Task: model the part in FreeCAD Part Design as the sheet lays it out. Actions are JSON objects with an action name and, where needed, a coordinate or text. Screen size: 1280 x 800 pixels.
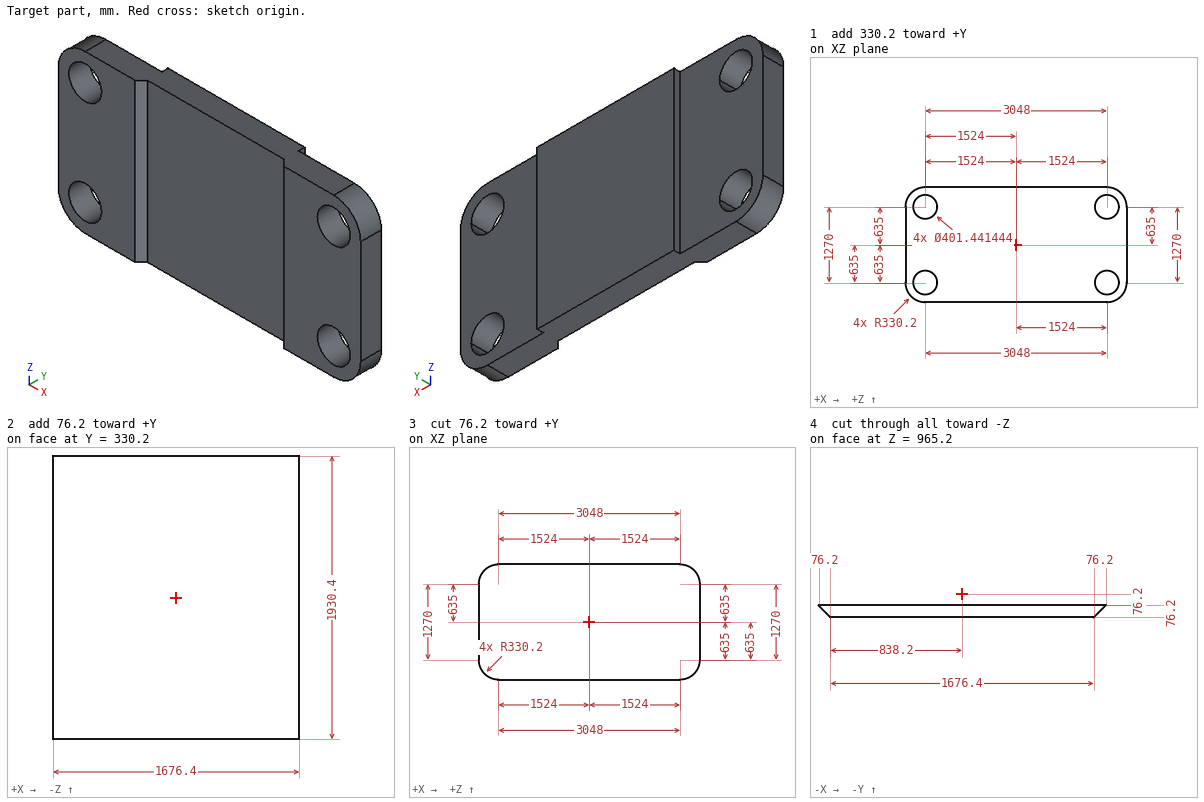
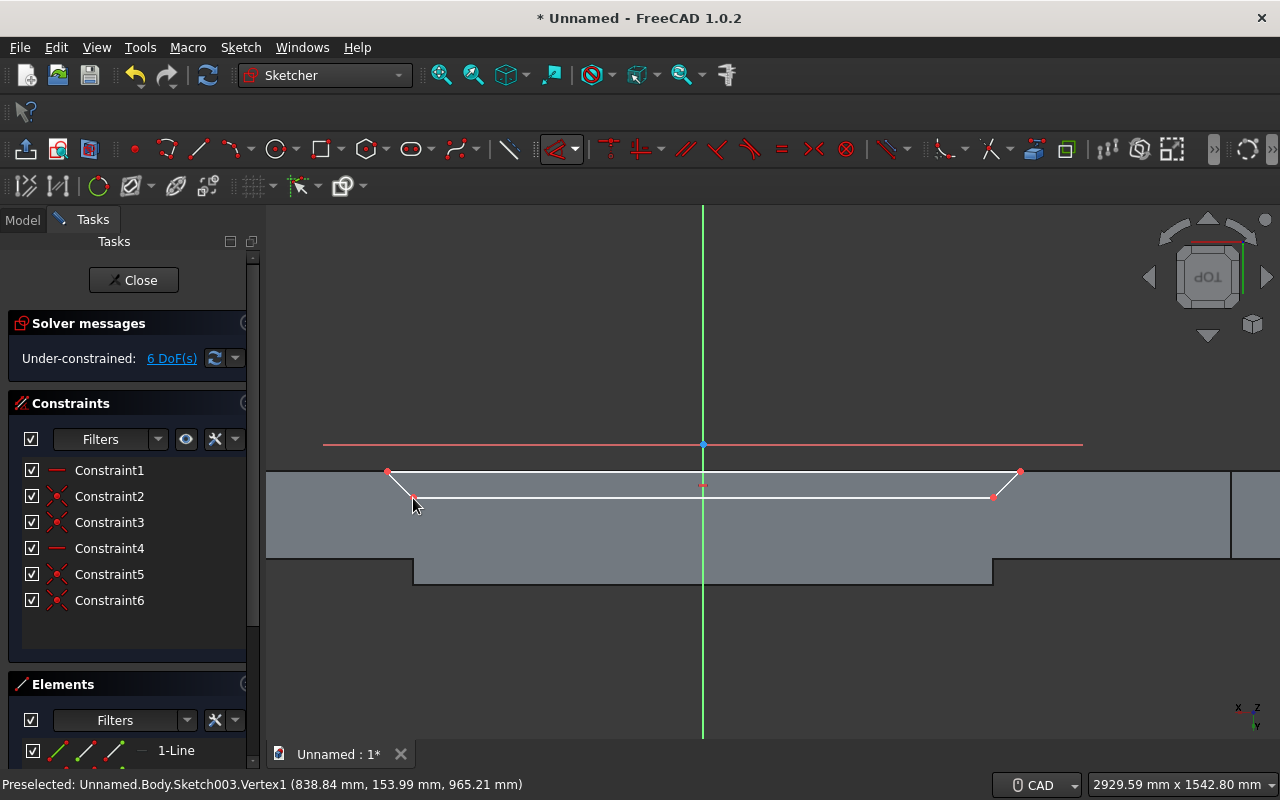
{"action": "scroll", "coordinate": [1020, 472], "scroll_direction": "up", "scroll_amount": 3}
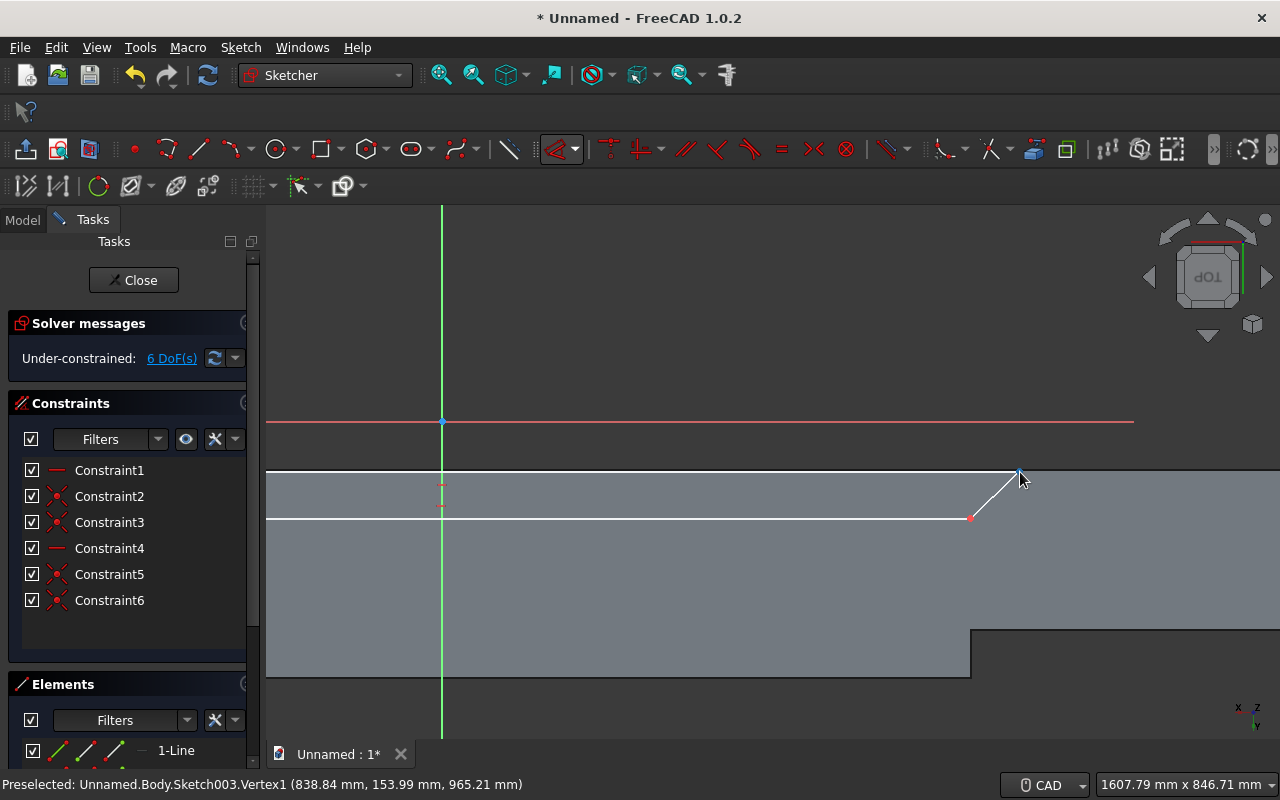
{"action": "left_click", "coordinate": [1019, 472]}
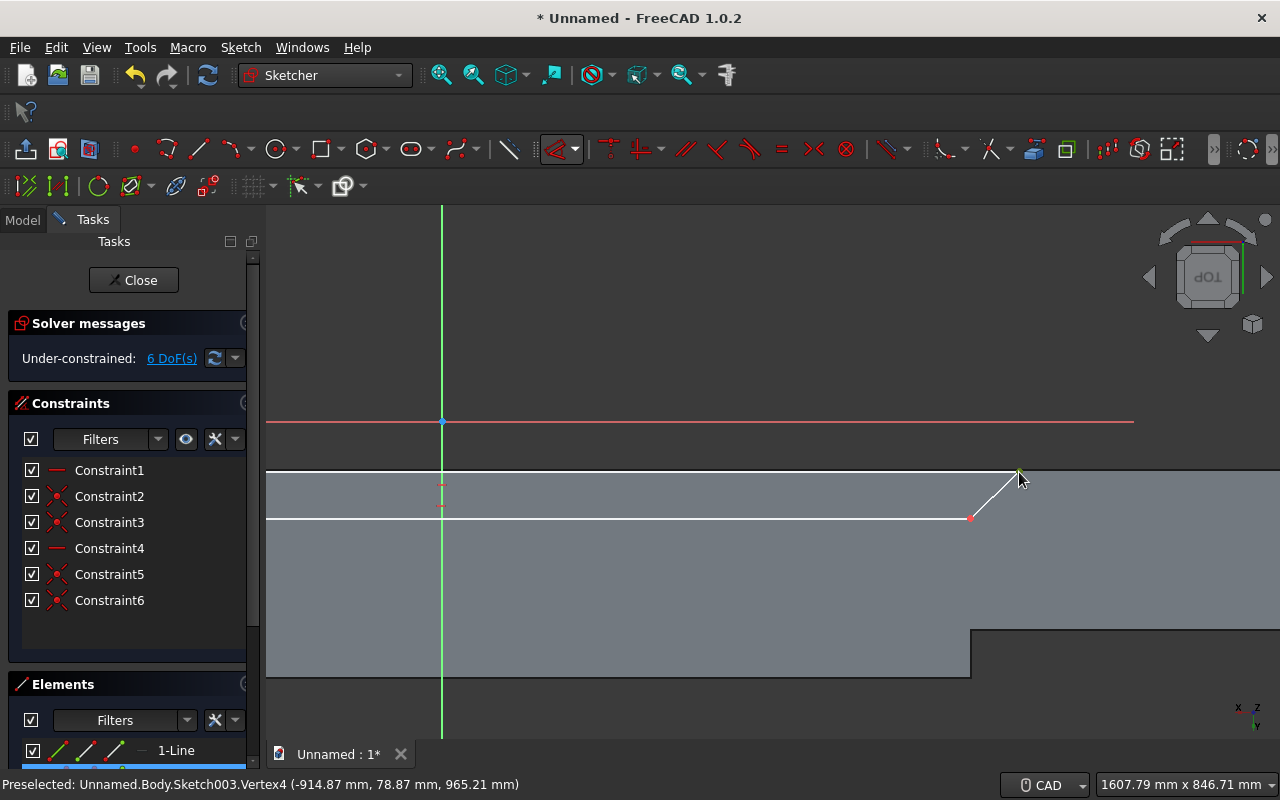
{"action": "key", "text": "i"}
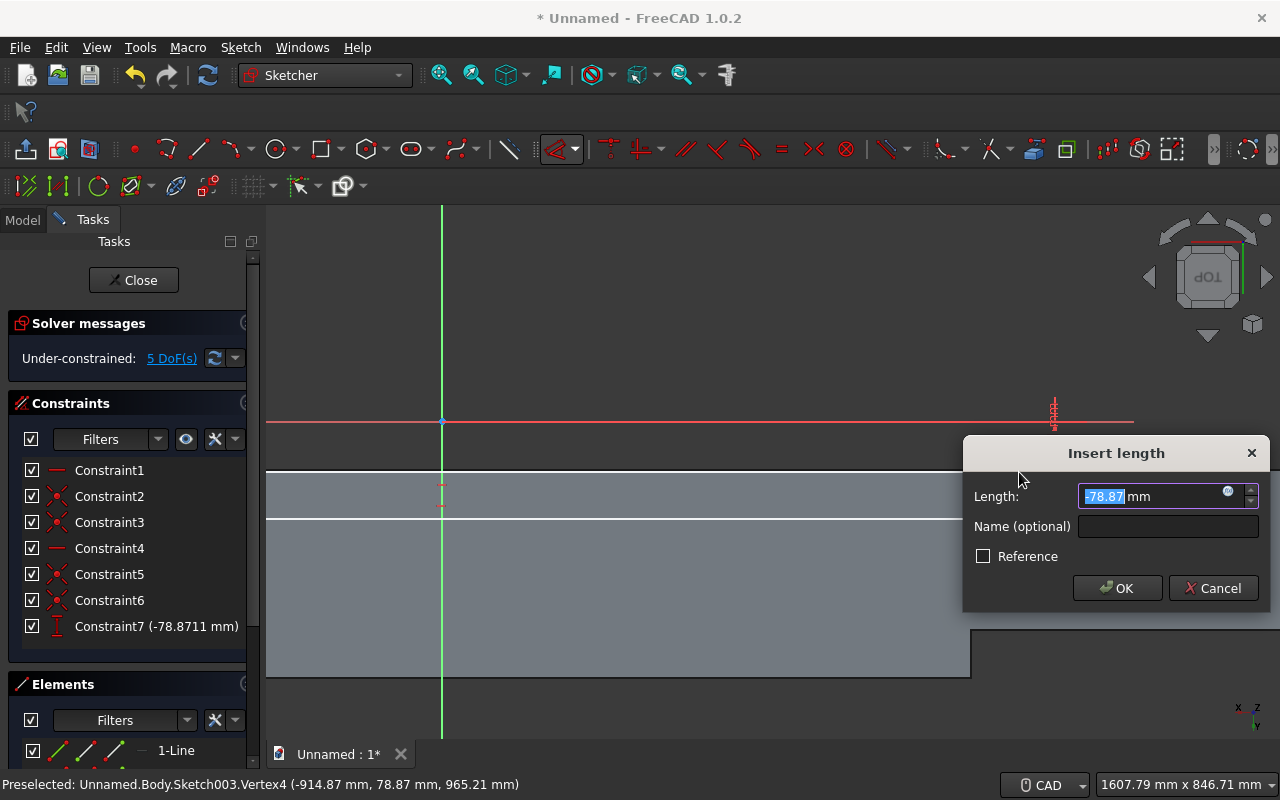
{"action": "type", "text": "-76.2"}
{"action": "key", "text": "Return"}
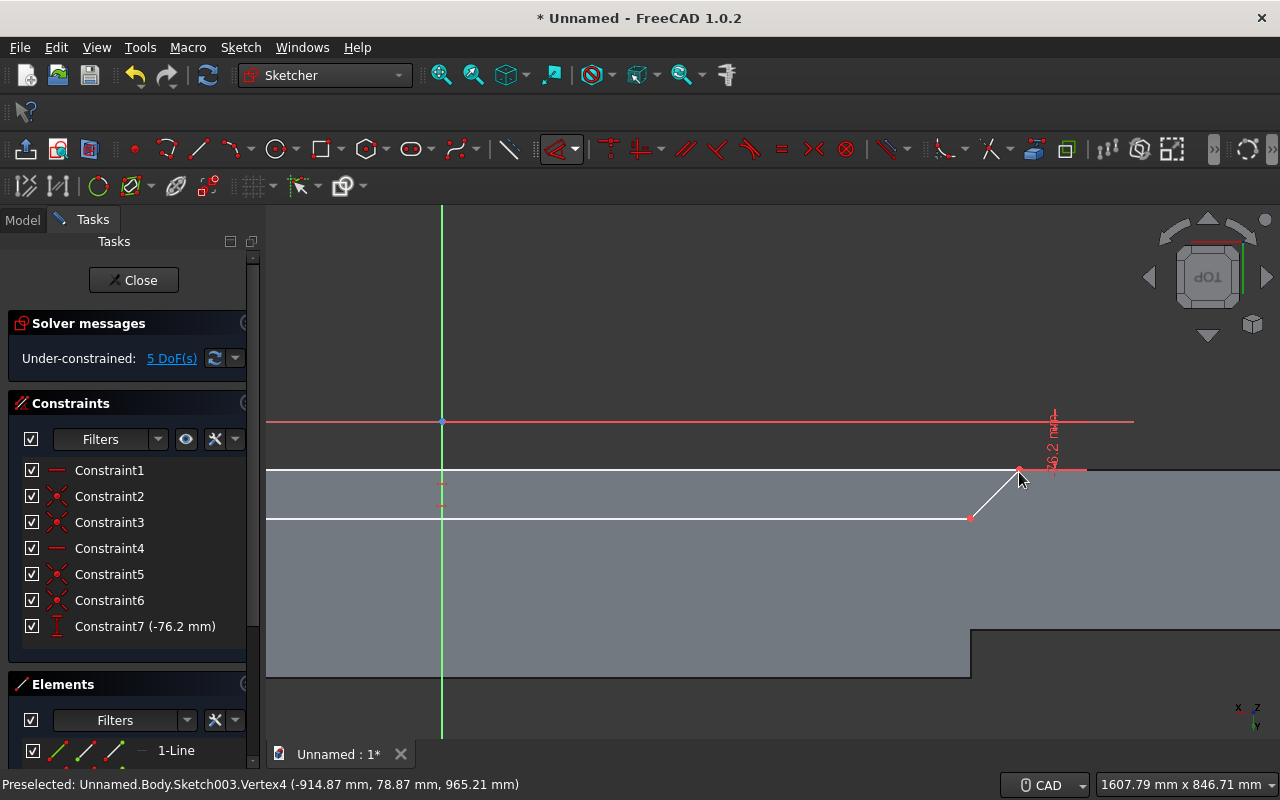
{"action": "left_click", "coordinate": [985, 504]}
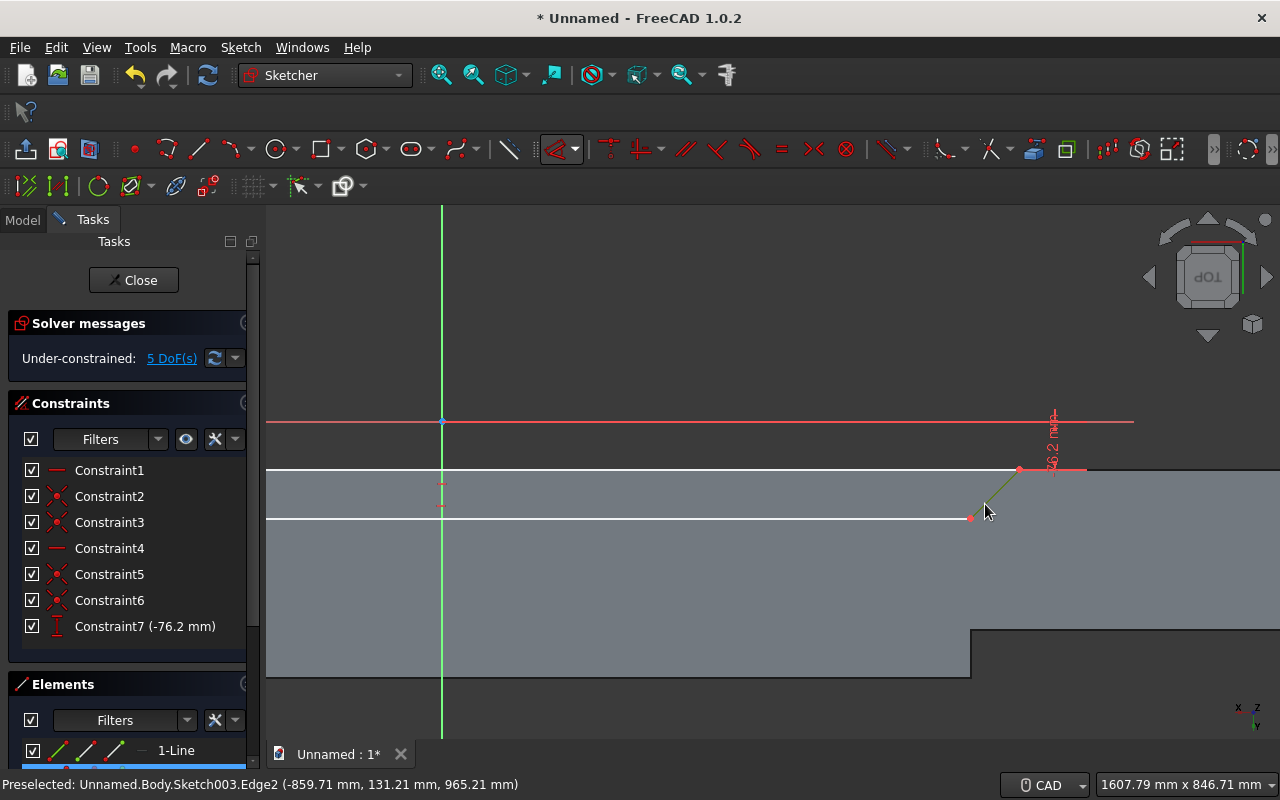
{"action": "key", "text": "l"}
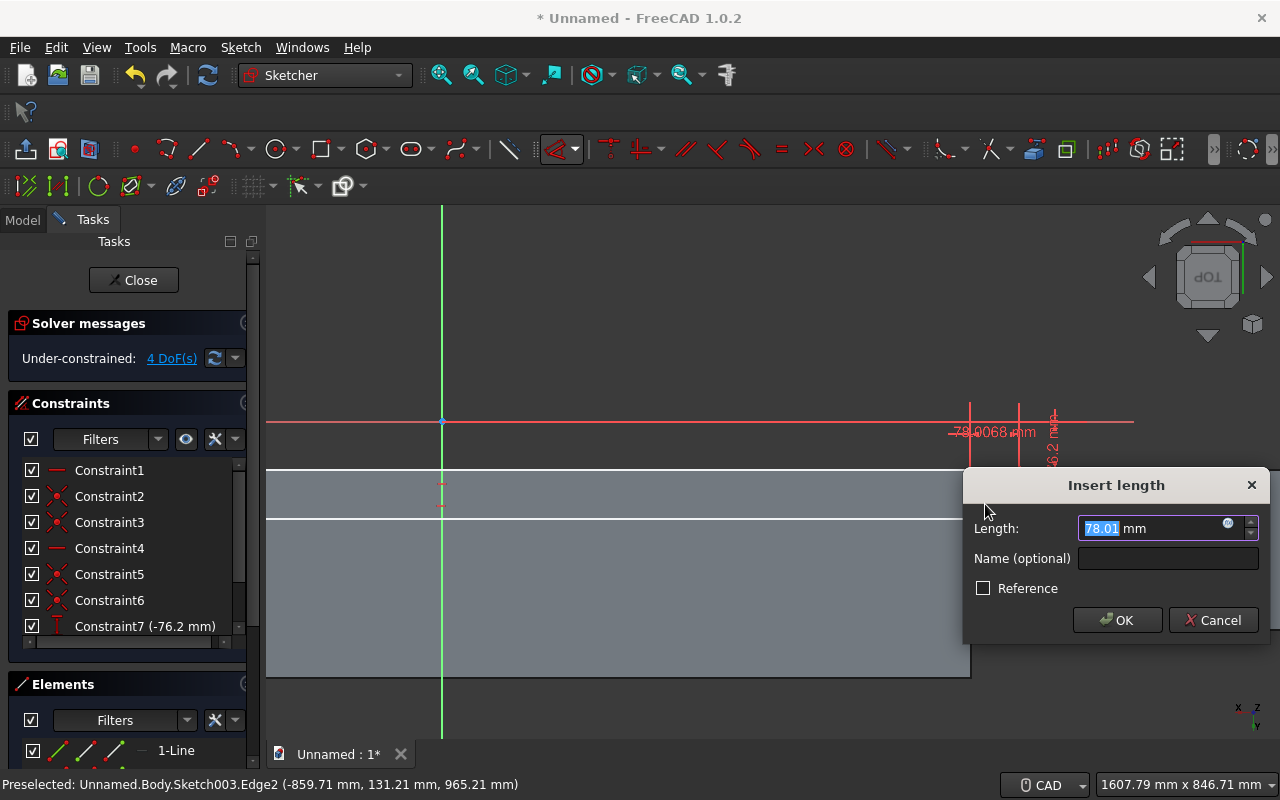
{"action": "type", "text": "76.2"}
{"action": "key", "text": "Return"}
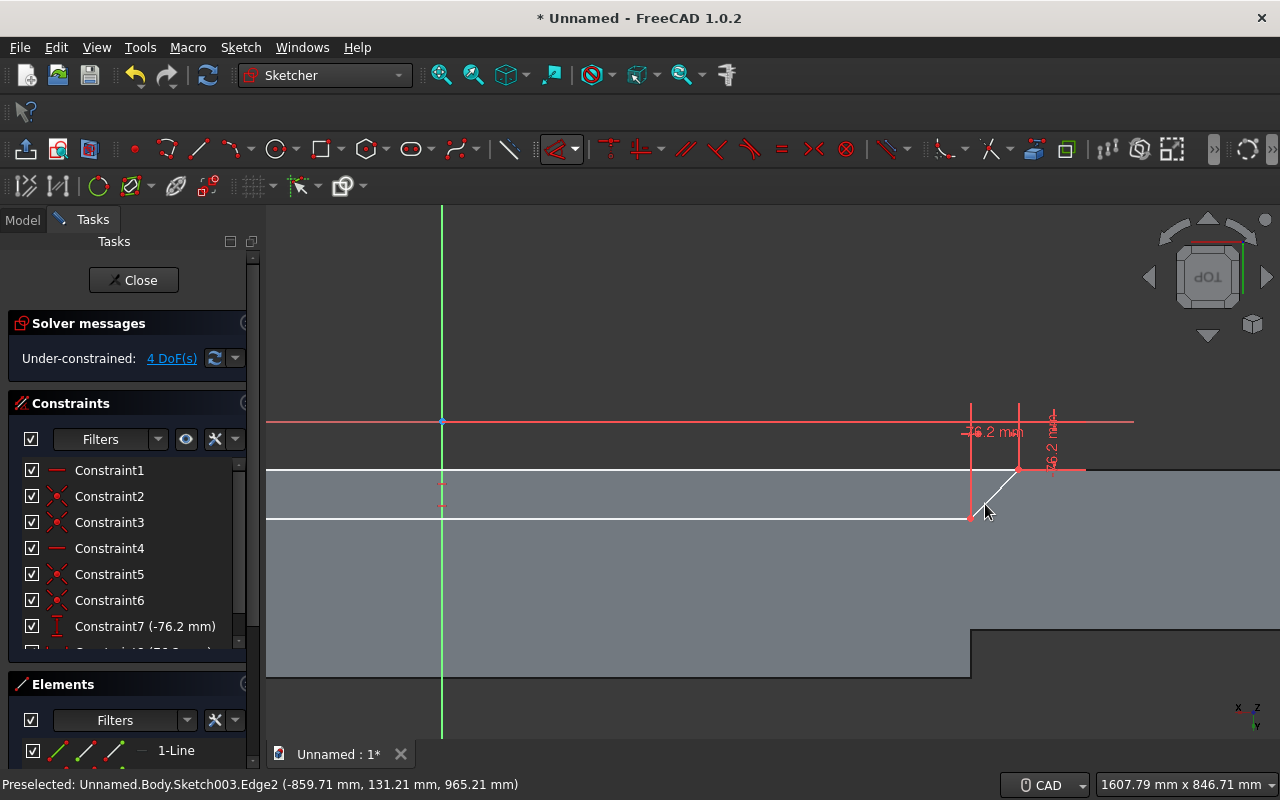
{"action": "left_click", "coordinate": [985, 504]}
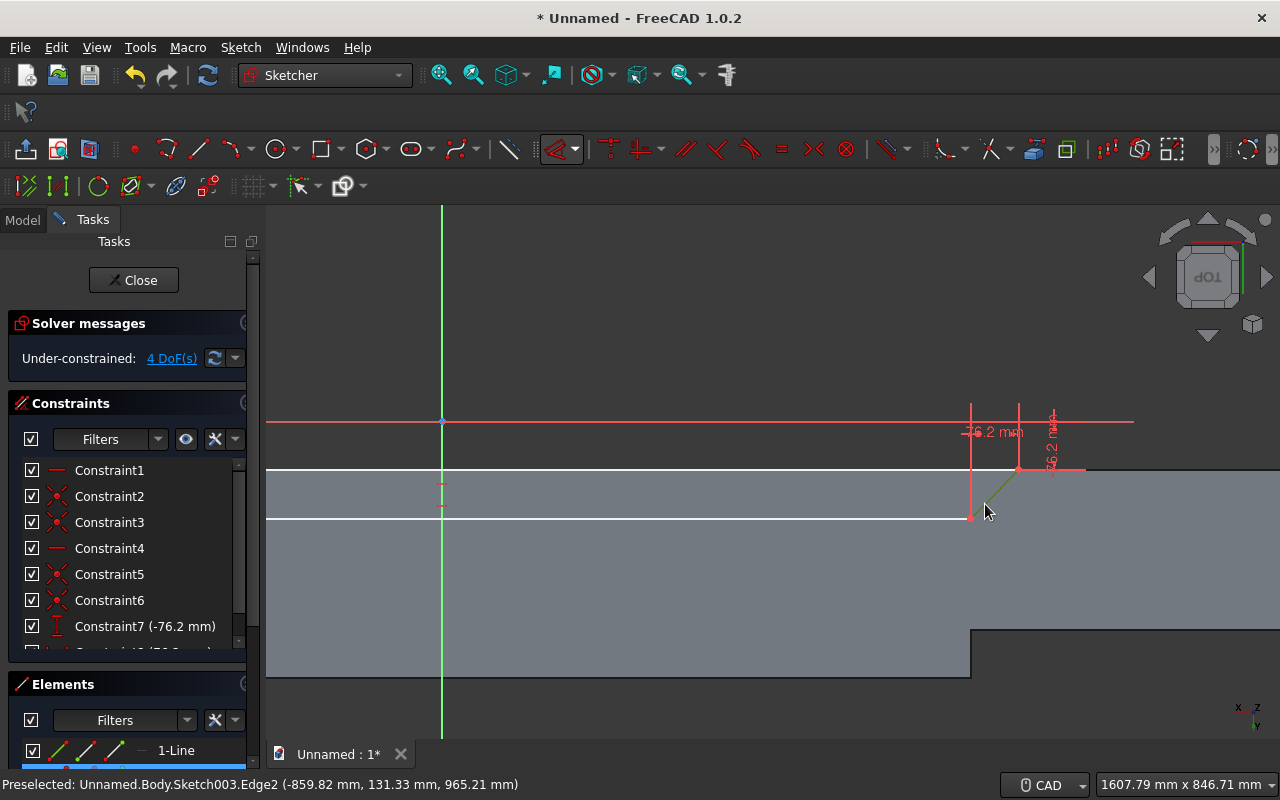
{"action": "key", "text": "i"}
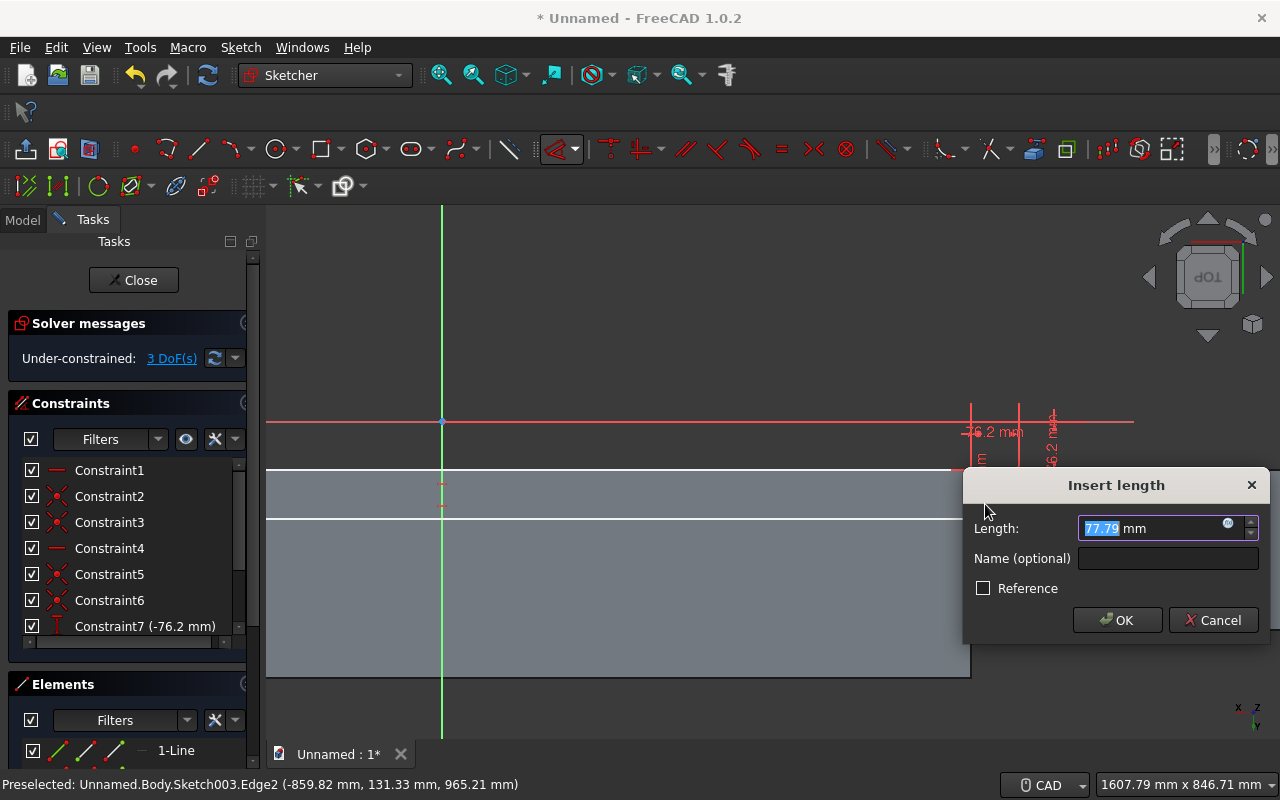
{"action": "type", "text": "76.2"}
{"action": "key", "text": "Return"}